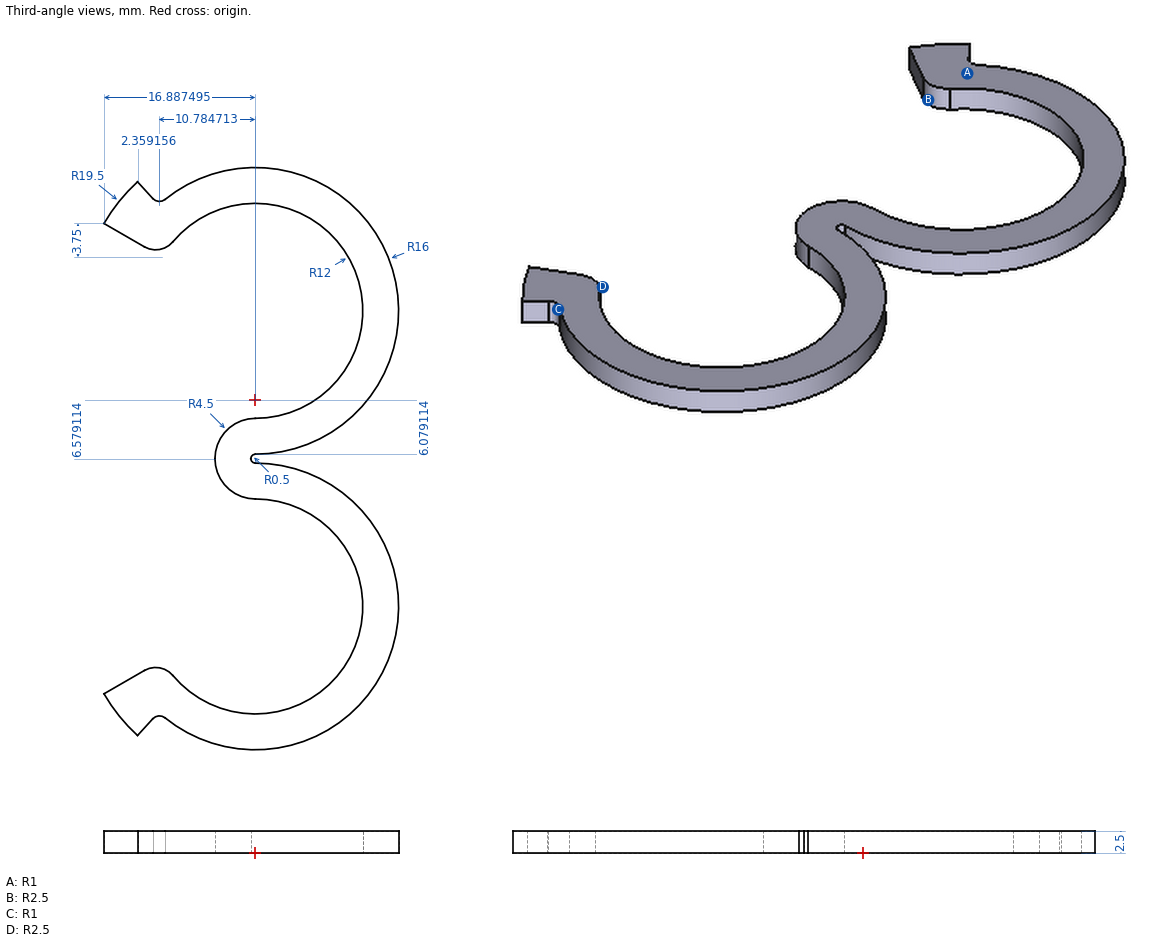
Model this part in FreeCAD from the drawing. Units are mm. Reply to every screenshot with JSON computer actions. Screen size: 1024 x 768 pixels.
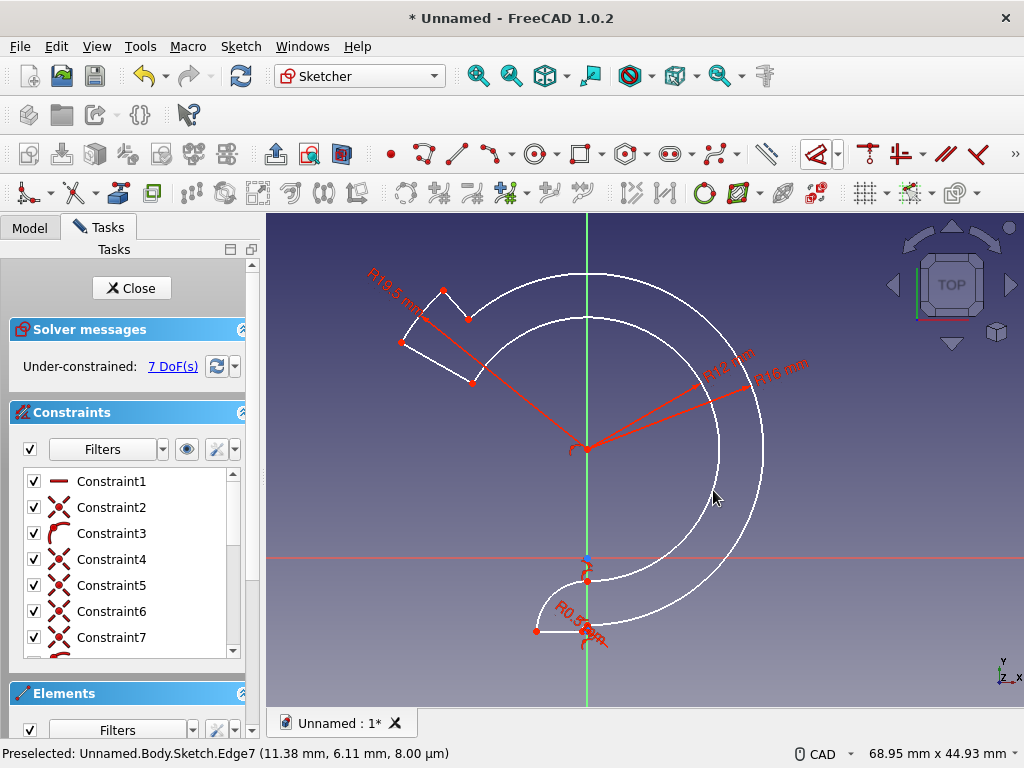
{"action": "left_click", "coordinate": [564, 587]}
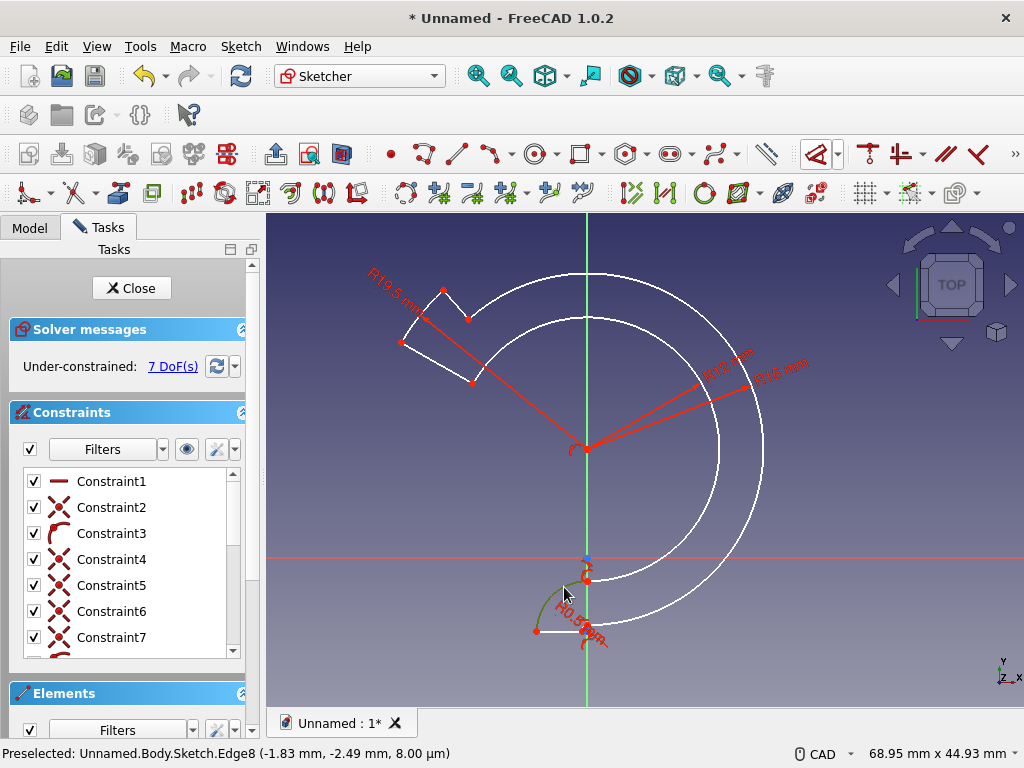
{"action": "key", "text": "k r"}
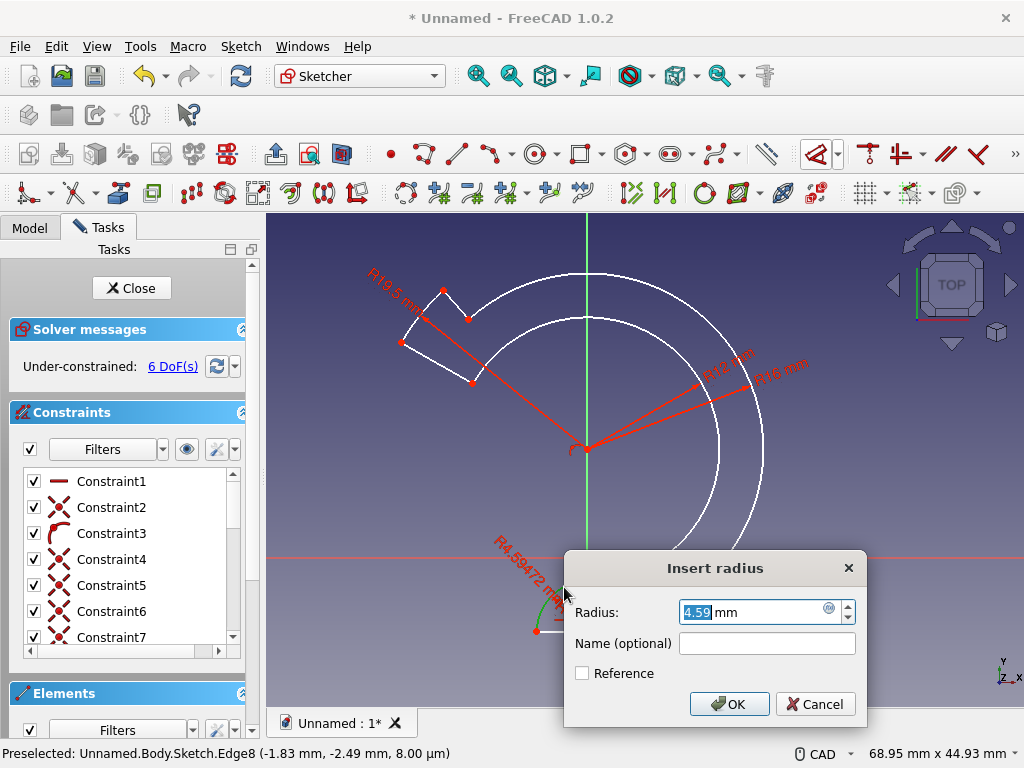
{"action": "type", "text": "4.5"}
{"action": "key", "text": "Return"}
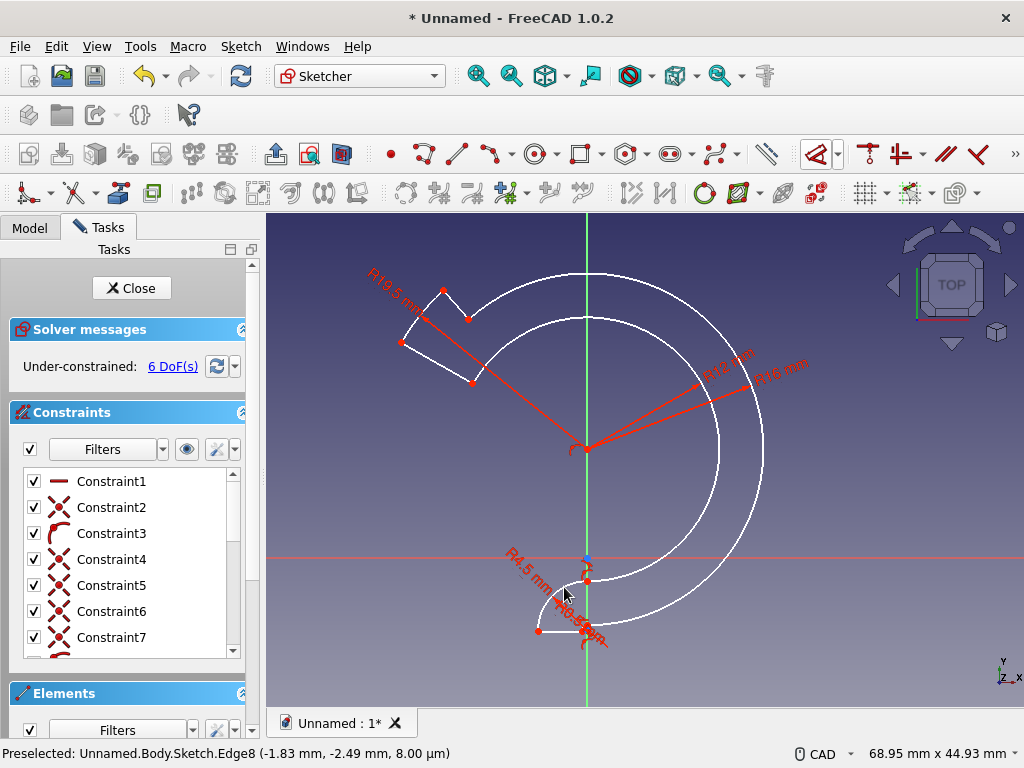
{"action": "left_click", "coordinate": [423, 355]}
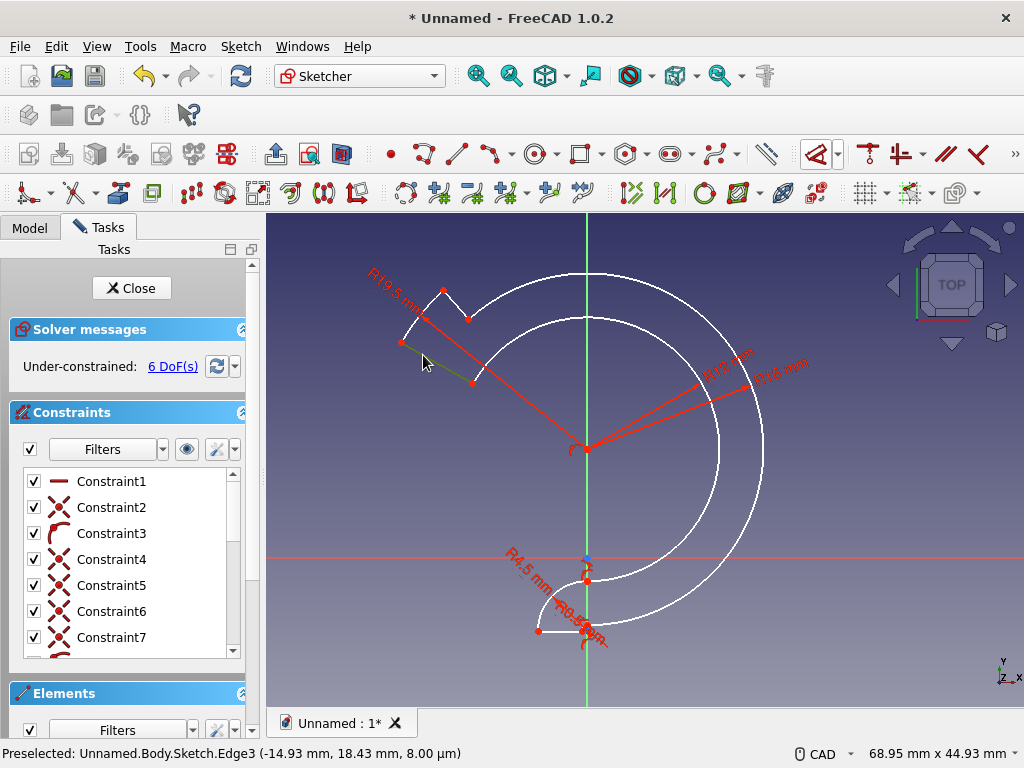
{"action": "key", "text": "i"}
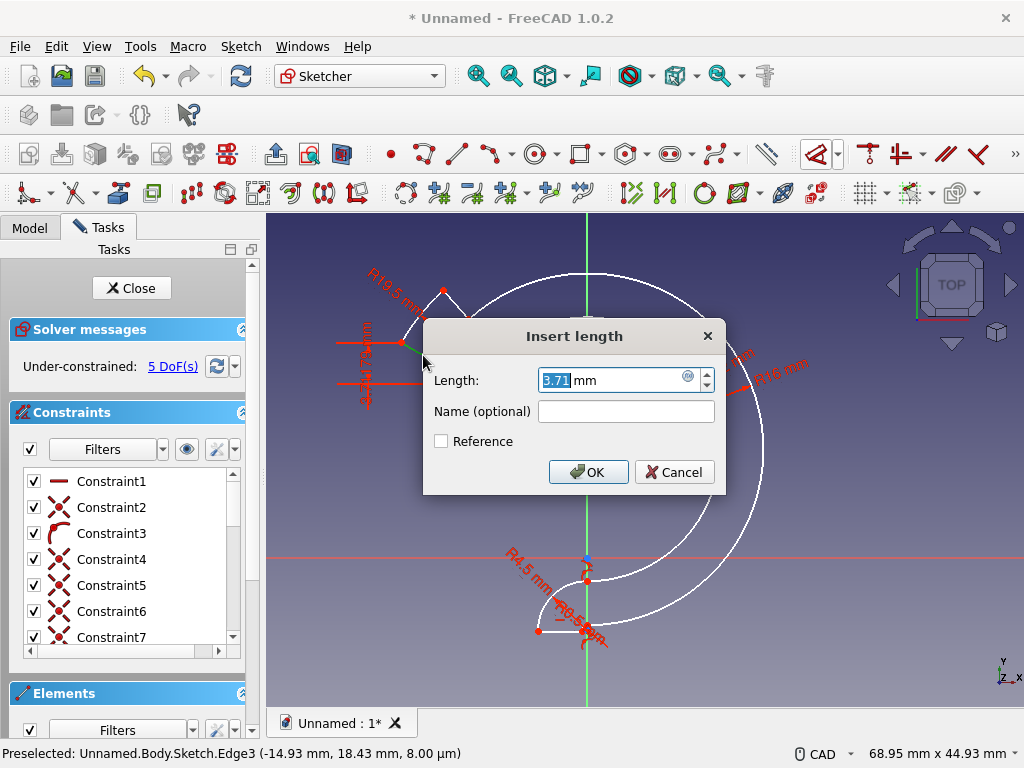
{"action": "type", "text": "3.75"}
{"action": "key", "text": "Return"}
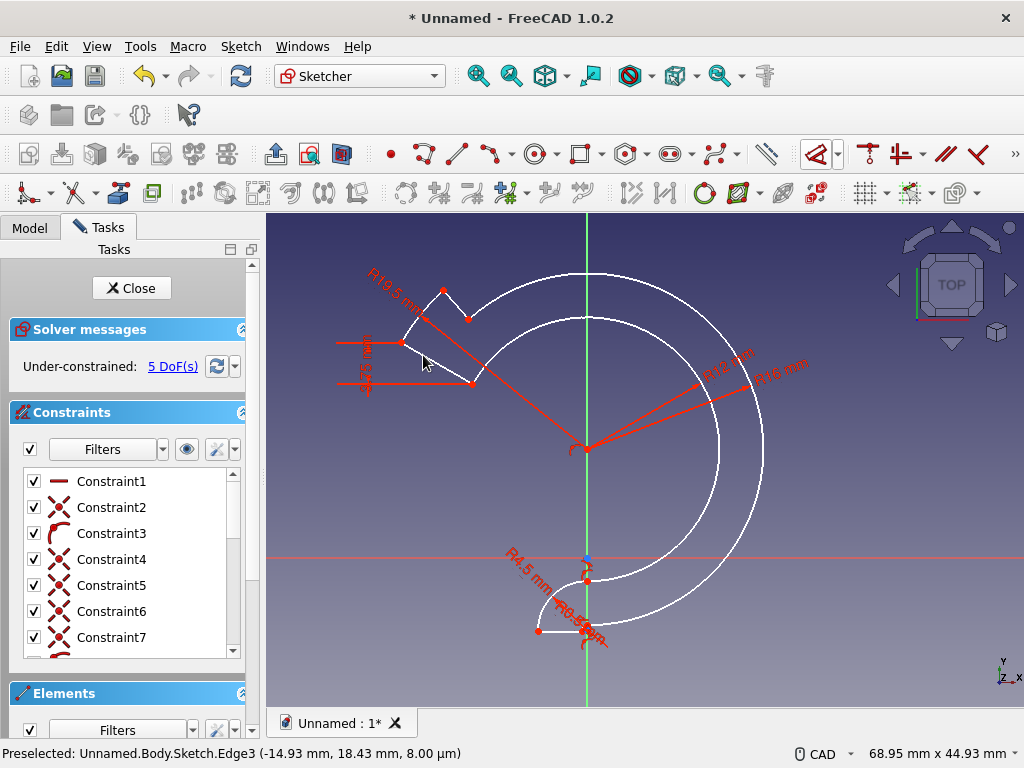
{"action": "left_click", "coordinate": [538, 632]}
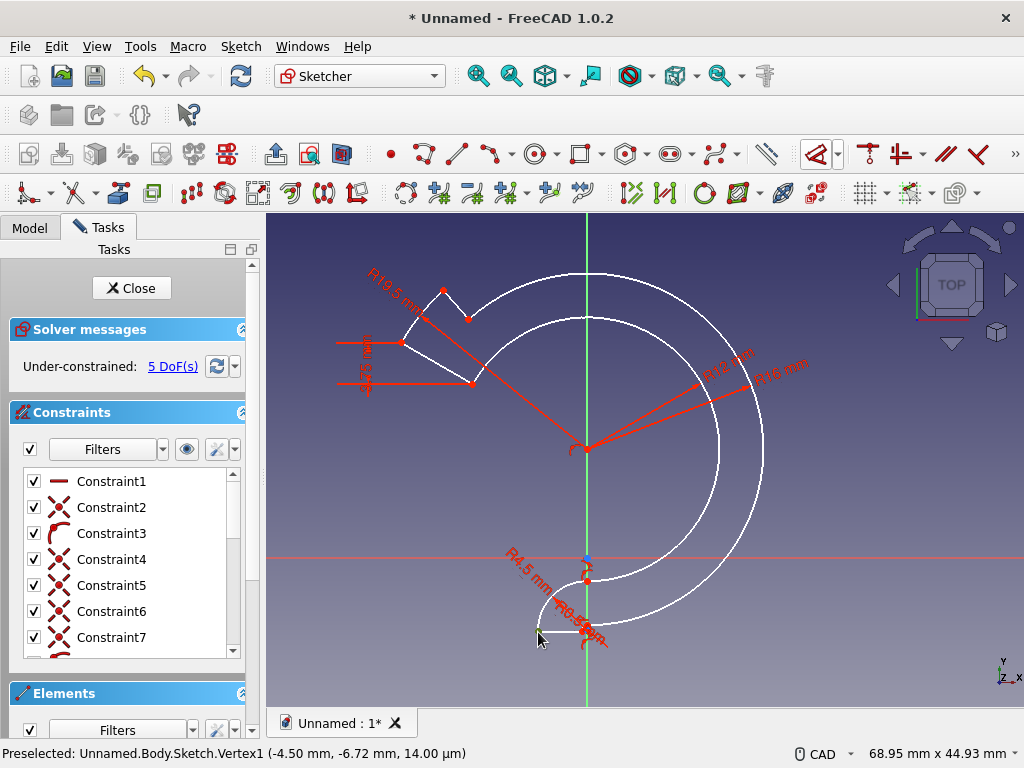
{"action": "left_click", "coordinate": [838, 154]}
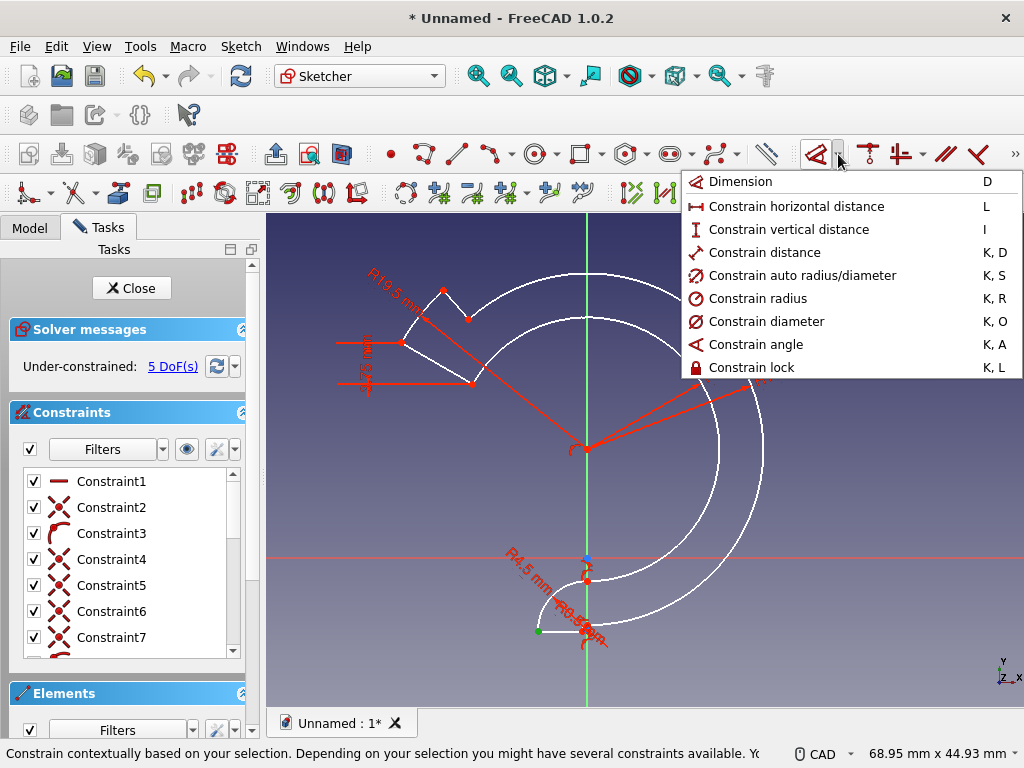
{"action": "left_click", "coordinate": [852, 230]}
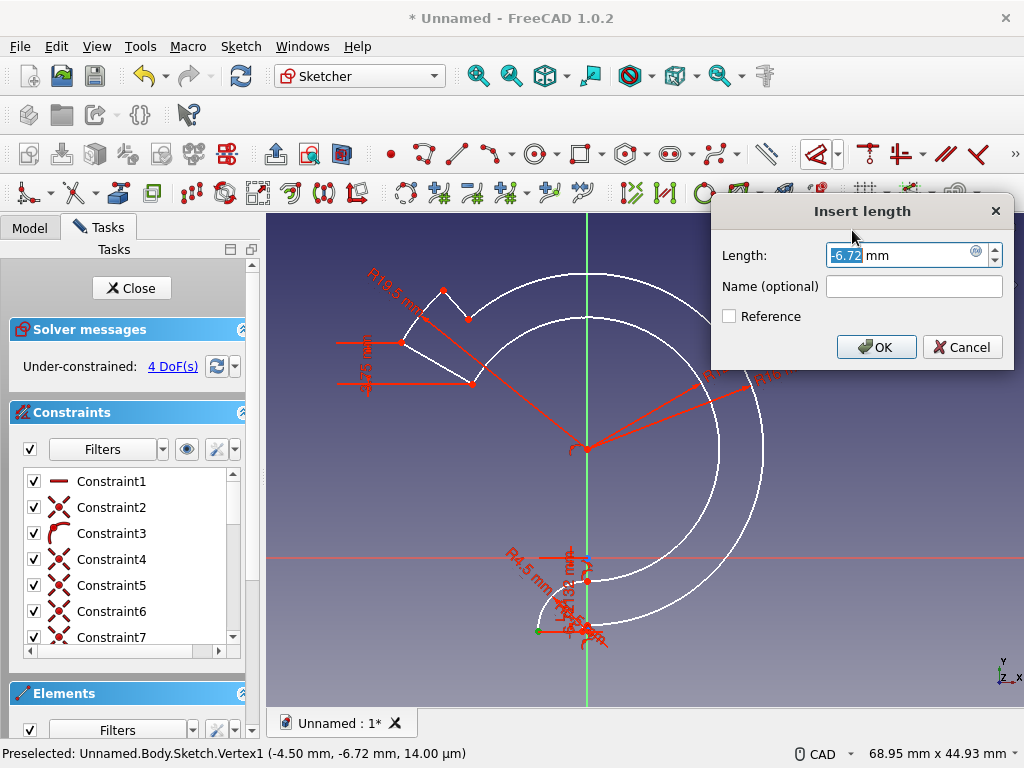
{"action": "type", "text": "-6.579114"}
{"action": "key", "text": "Return"}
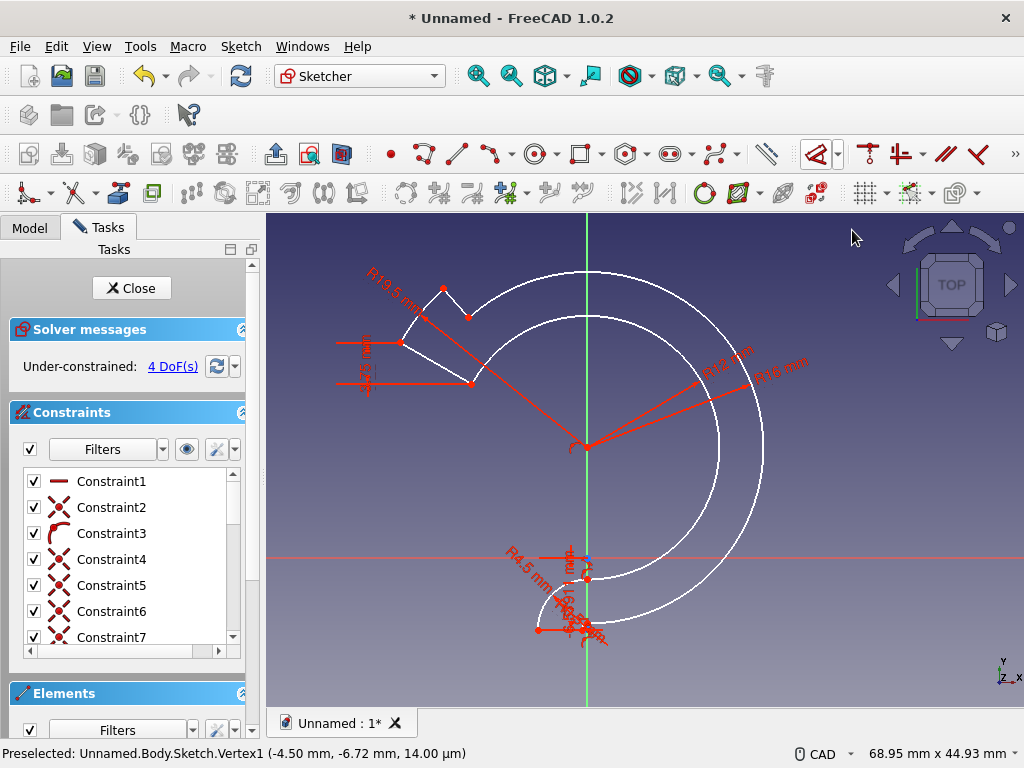
{"action": "scroll", "coordinate": [587, 624], "scroll_direction": "up", "scroll_amount": 4}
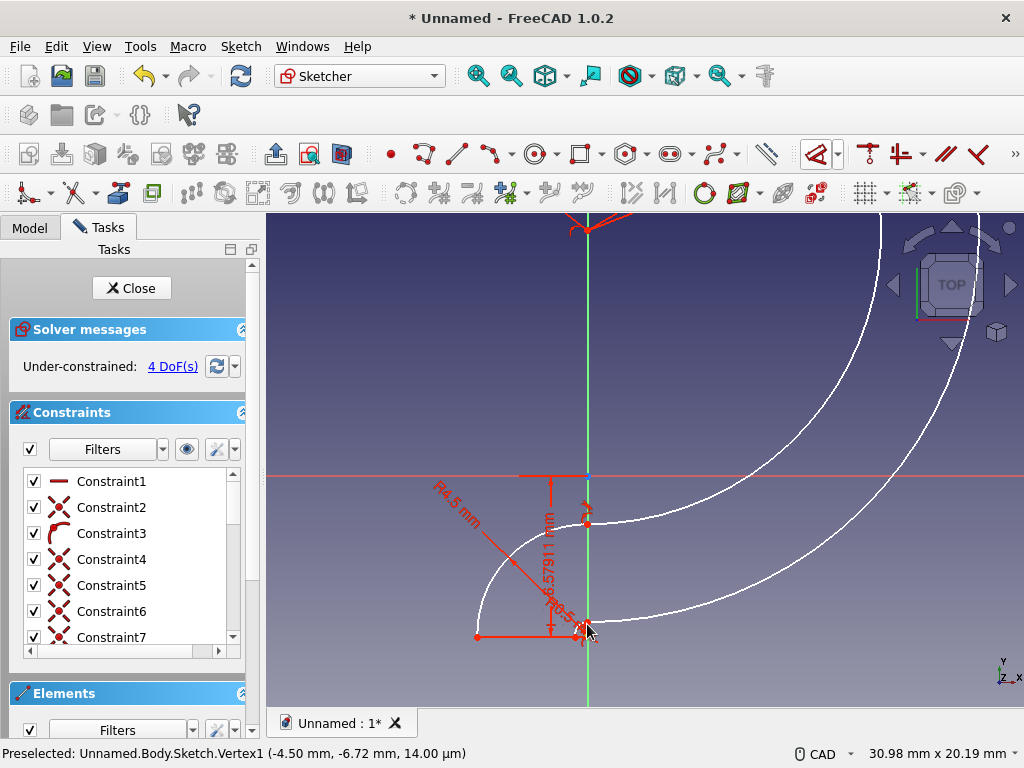
{"action": "left_click", "coordinate": [588, 622]}